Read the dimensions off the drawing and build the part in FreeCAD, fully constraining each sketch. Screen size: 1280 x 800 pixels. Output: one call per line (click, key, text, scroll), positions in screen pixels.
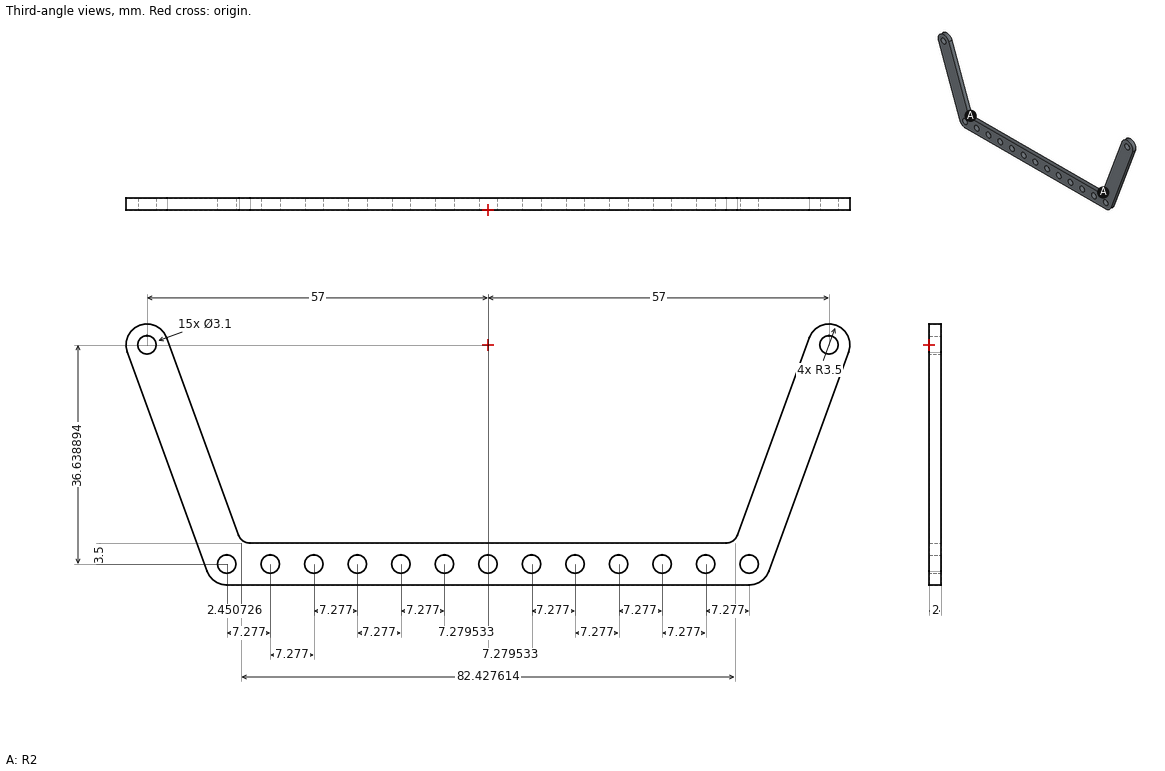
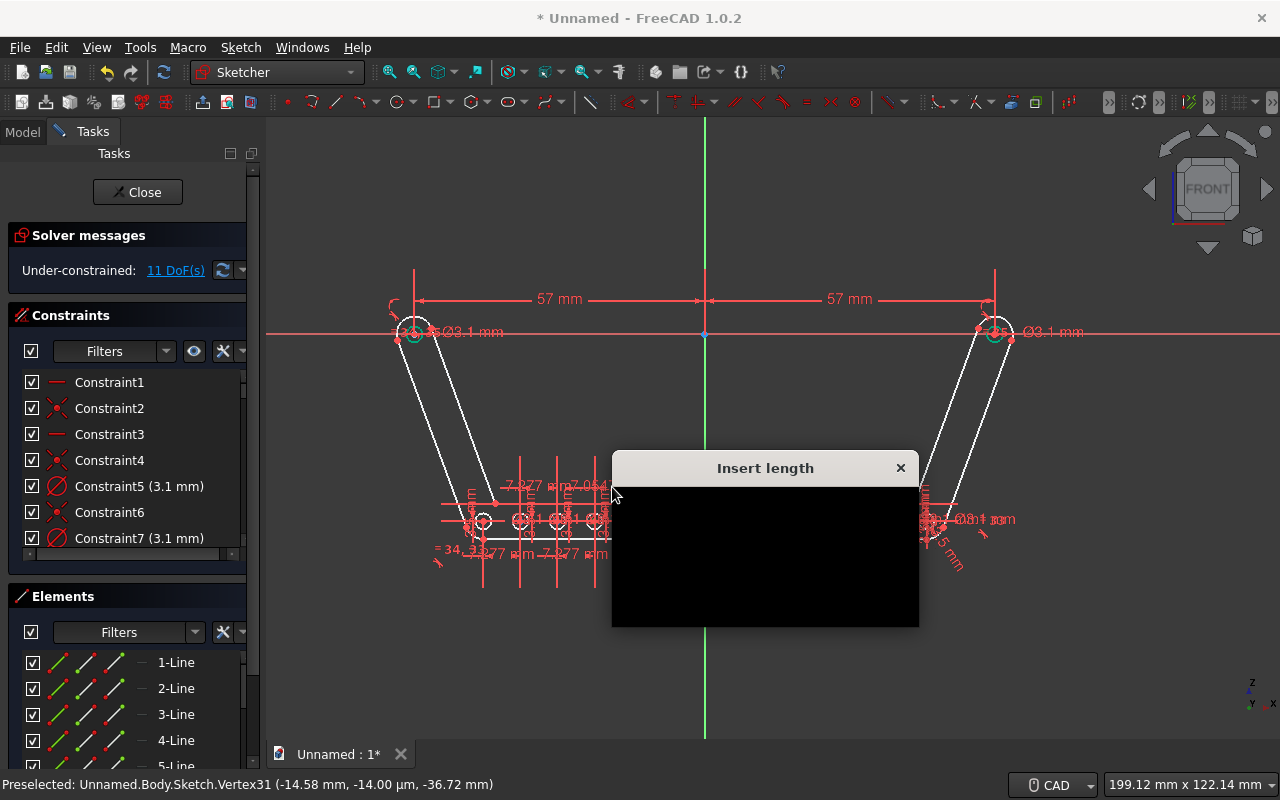
text(7.277)
key(Return)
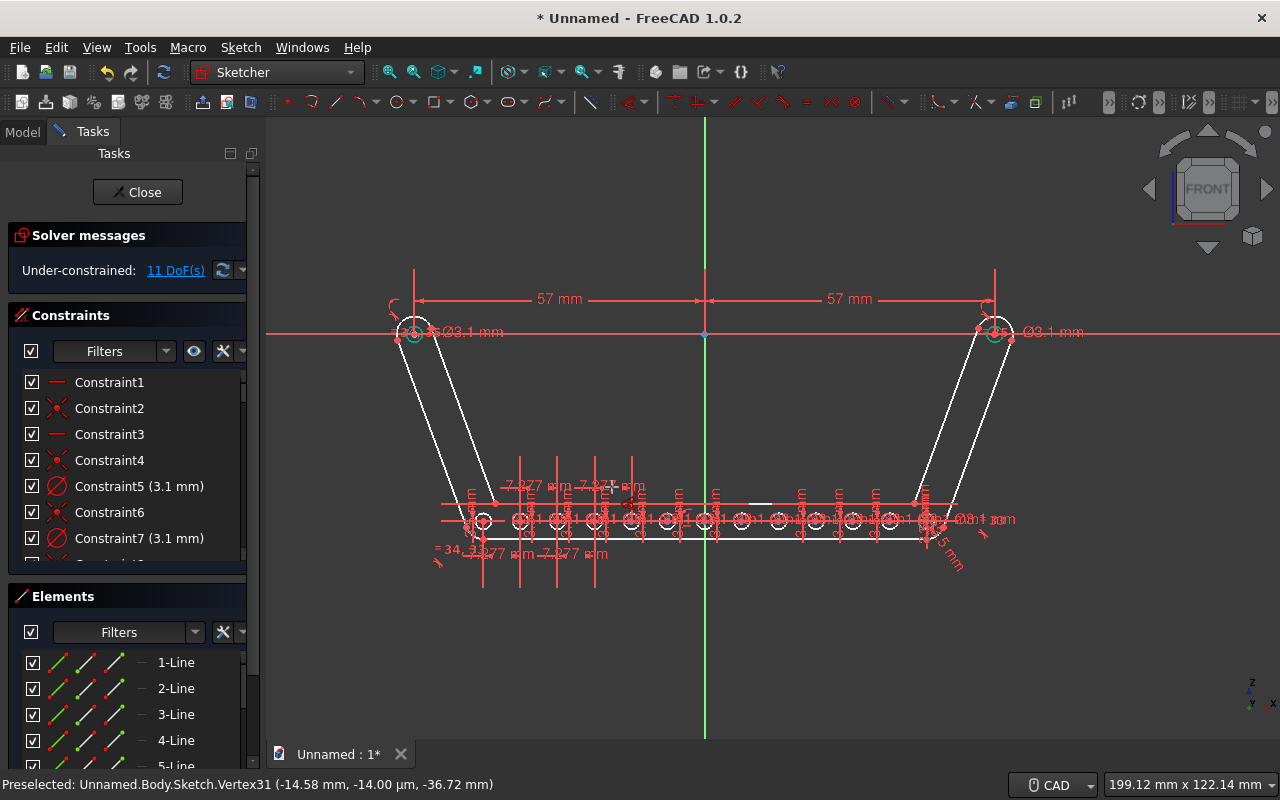
click(632, 521)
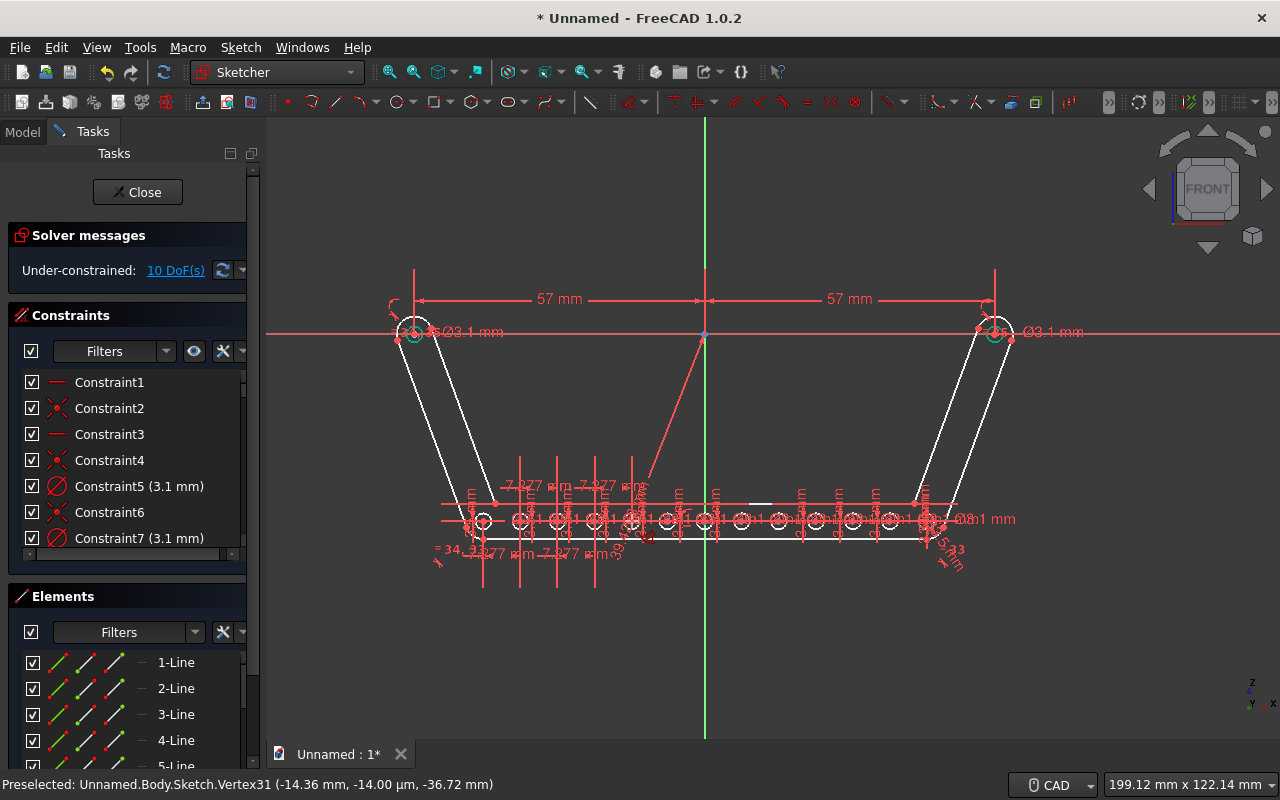
click(667, 521)
click(650, 555)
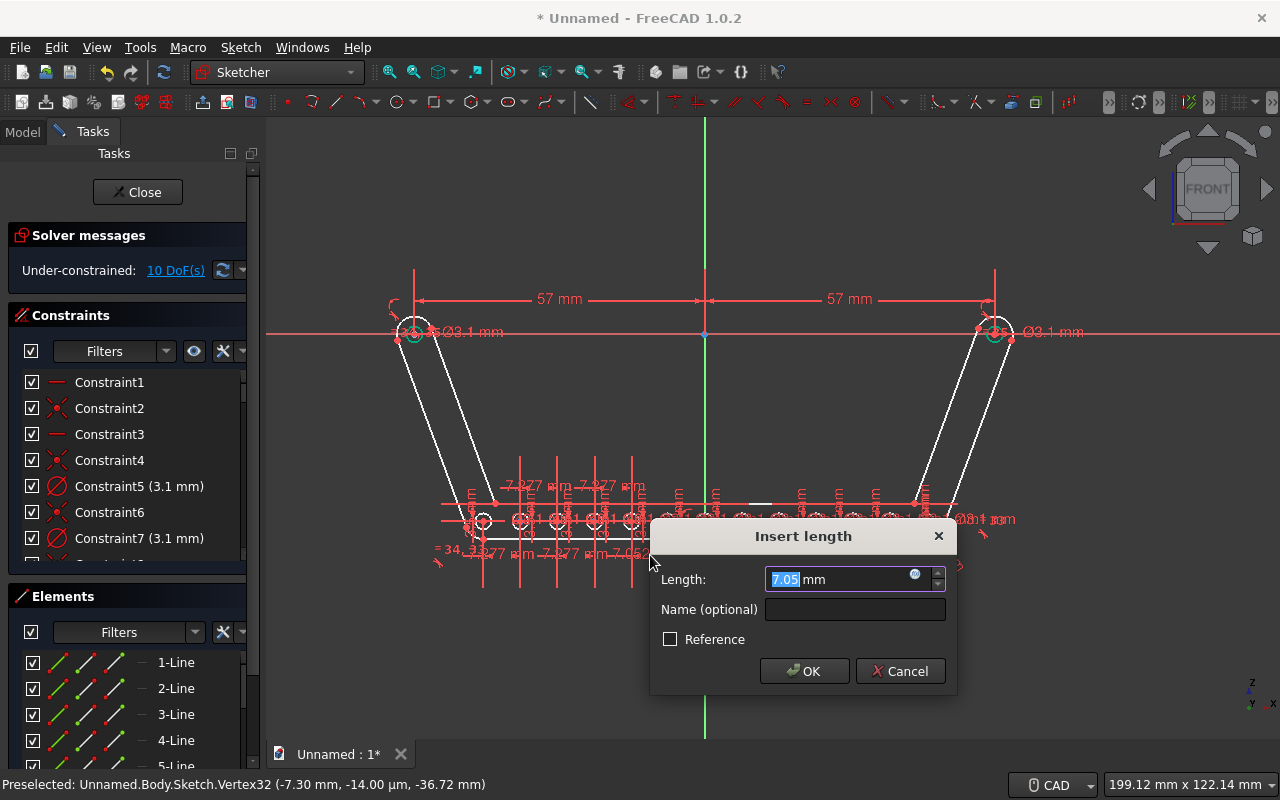
text(7.277)
key(Return)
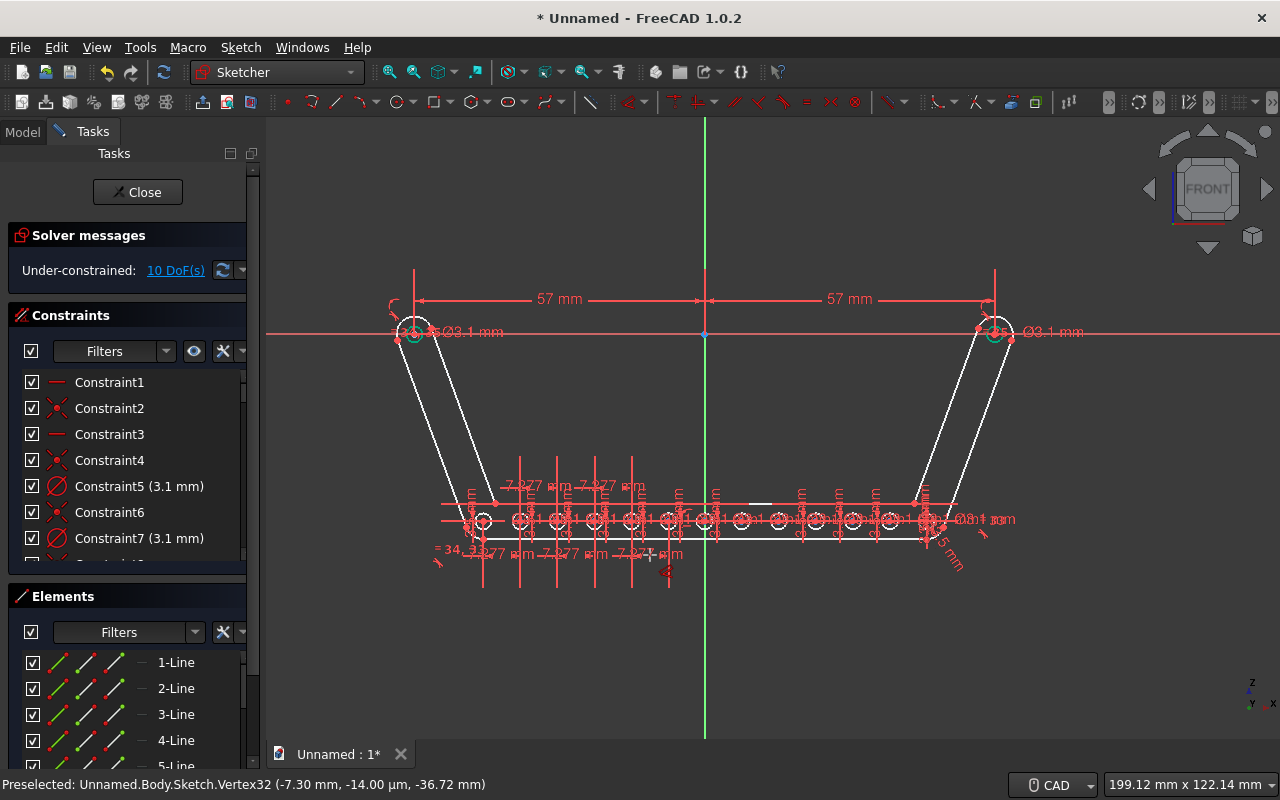
click(742, 521)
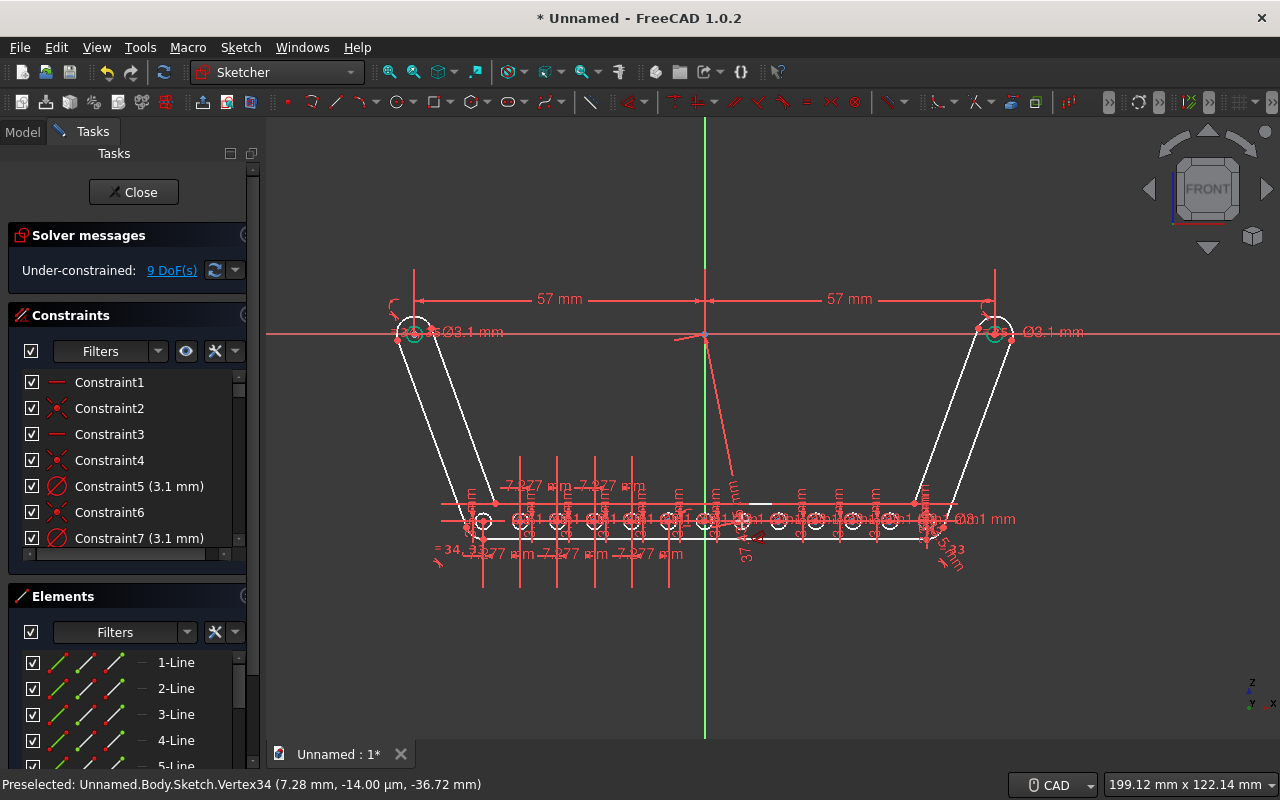
click(779, 521)
click(760, 555)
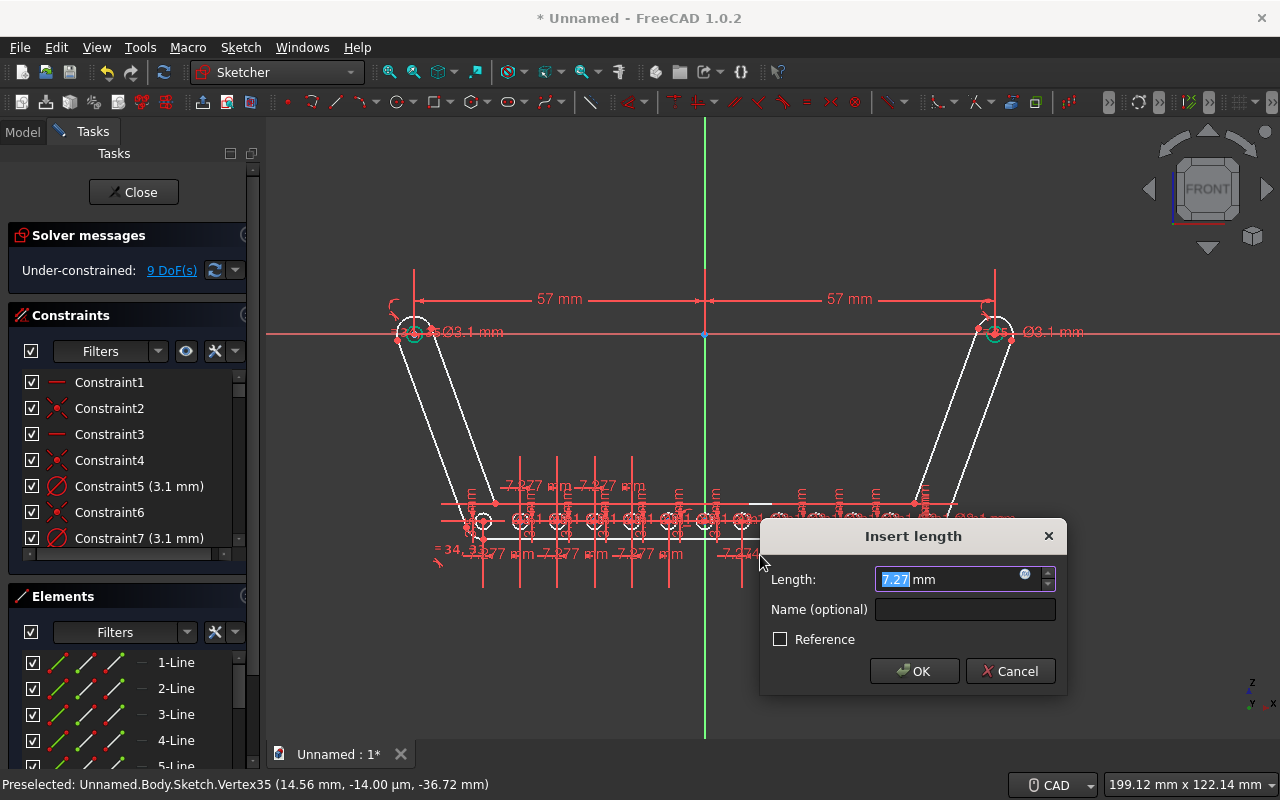
text(7.277)
key(Return)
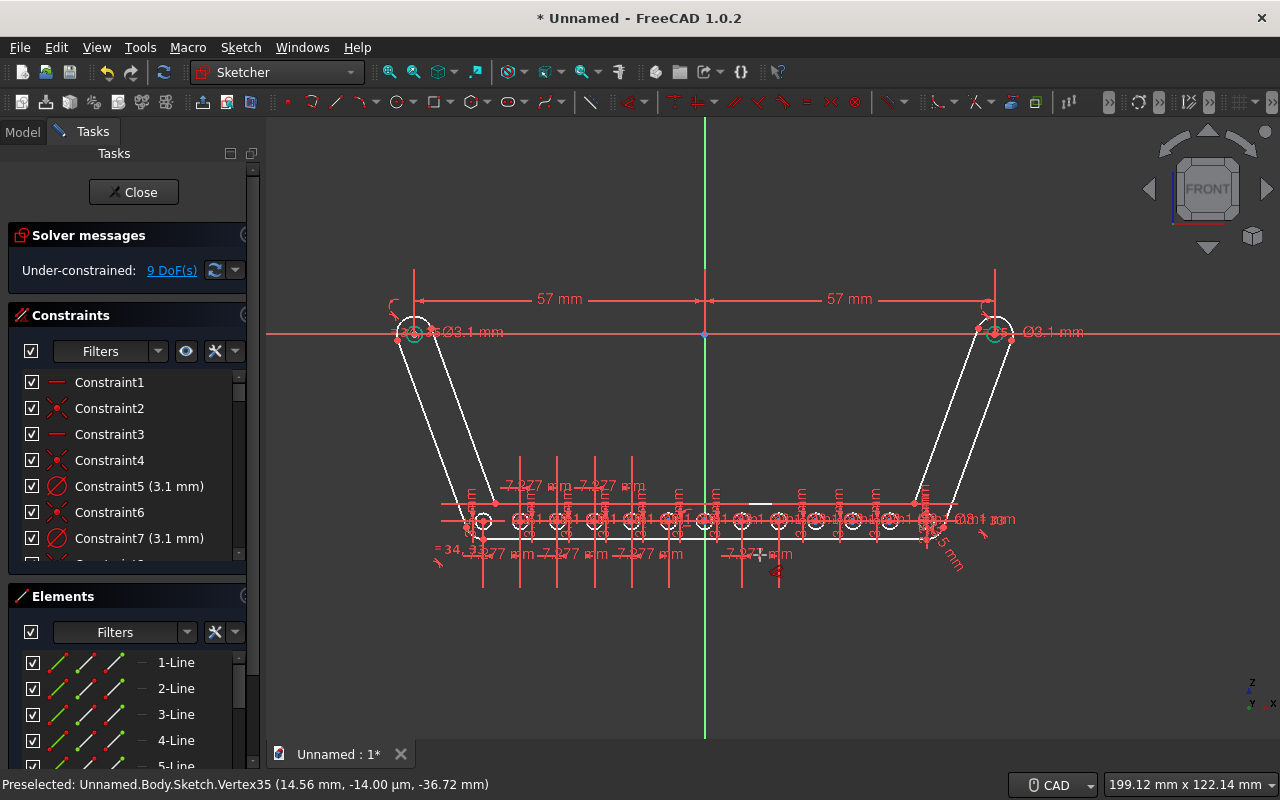
click(779, 521)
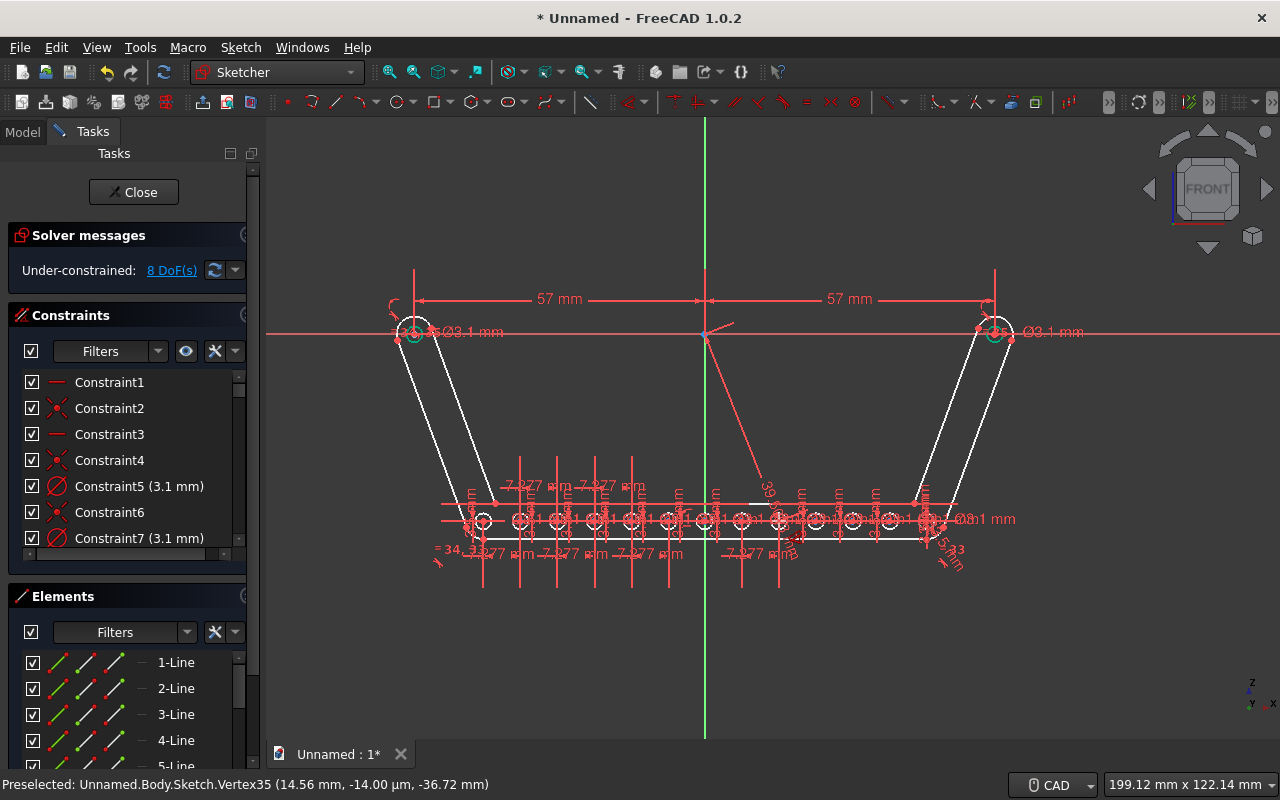
click(816, 521)
click(797, 487)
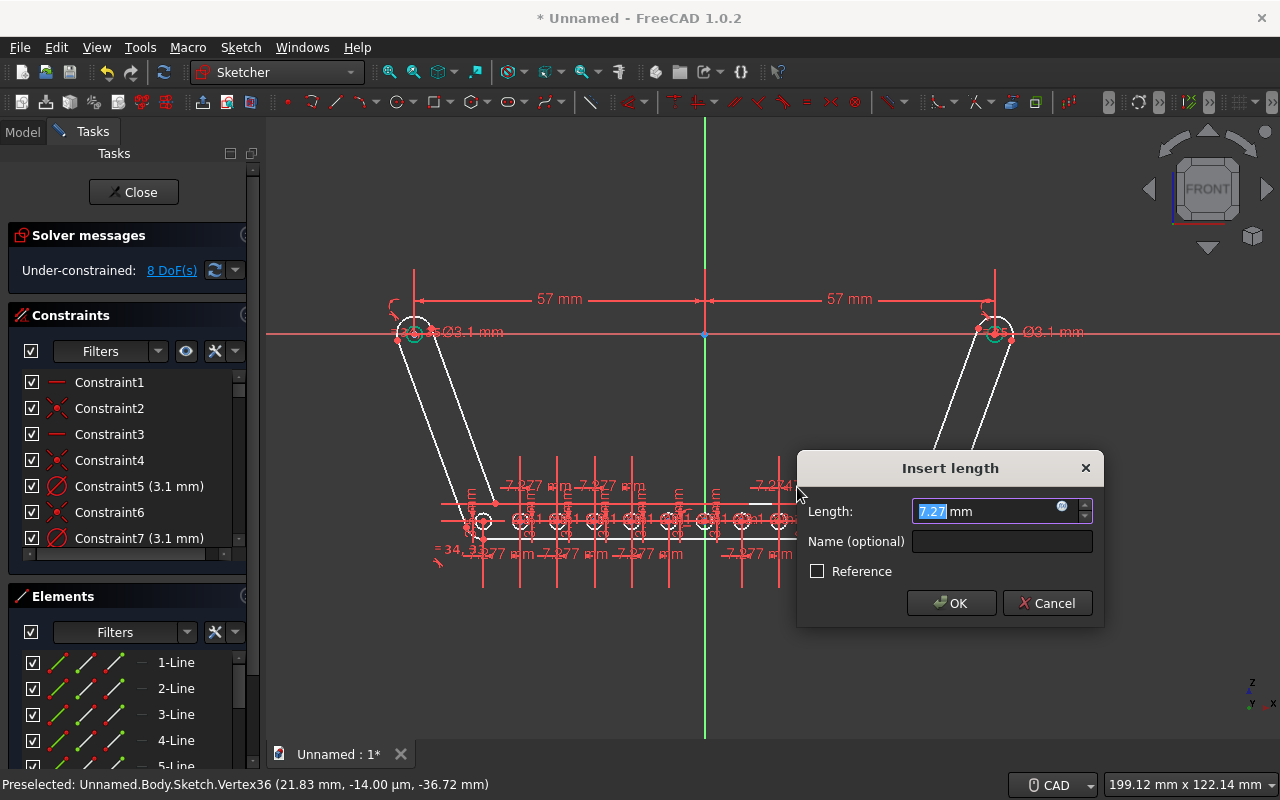
text(7.277)
key(Return)